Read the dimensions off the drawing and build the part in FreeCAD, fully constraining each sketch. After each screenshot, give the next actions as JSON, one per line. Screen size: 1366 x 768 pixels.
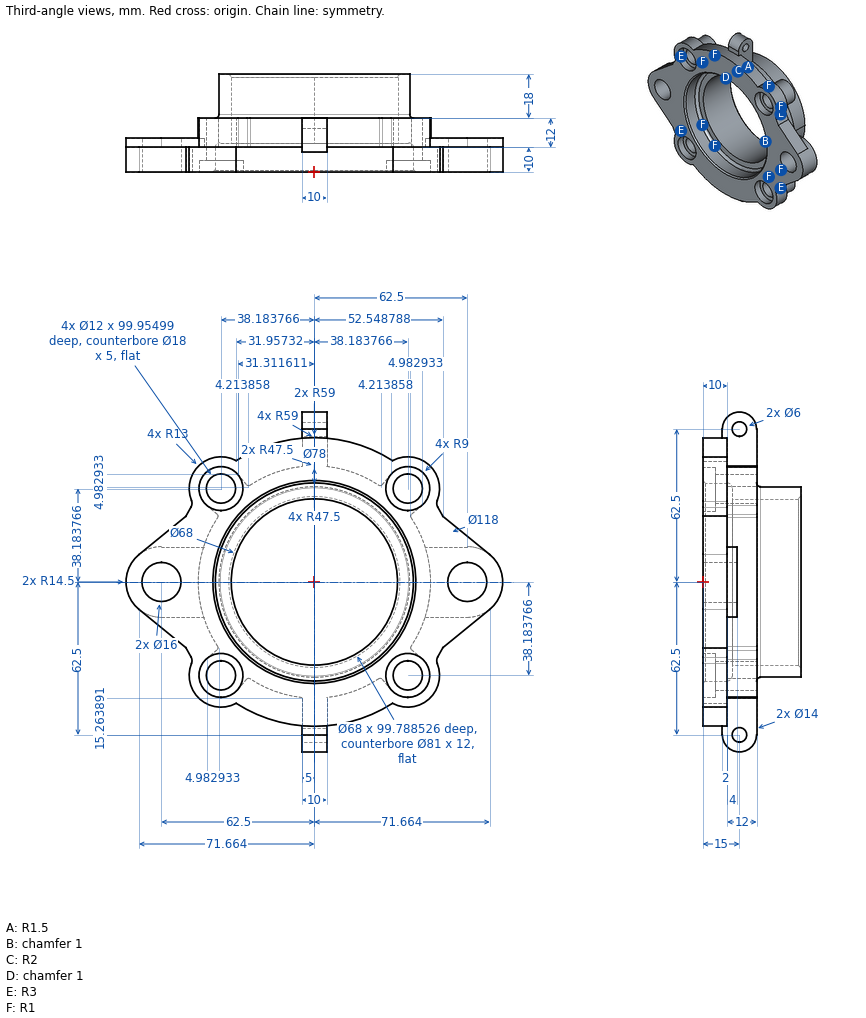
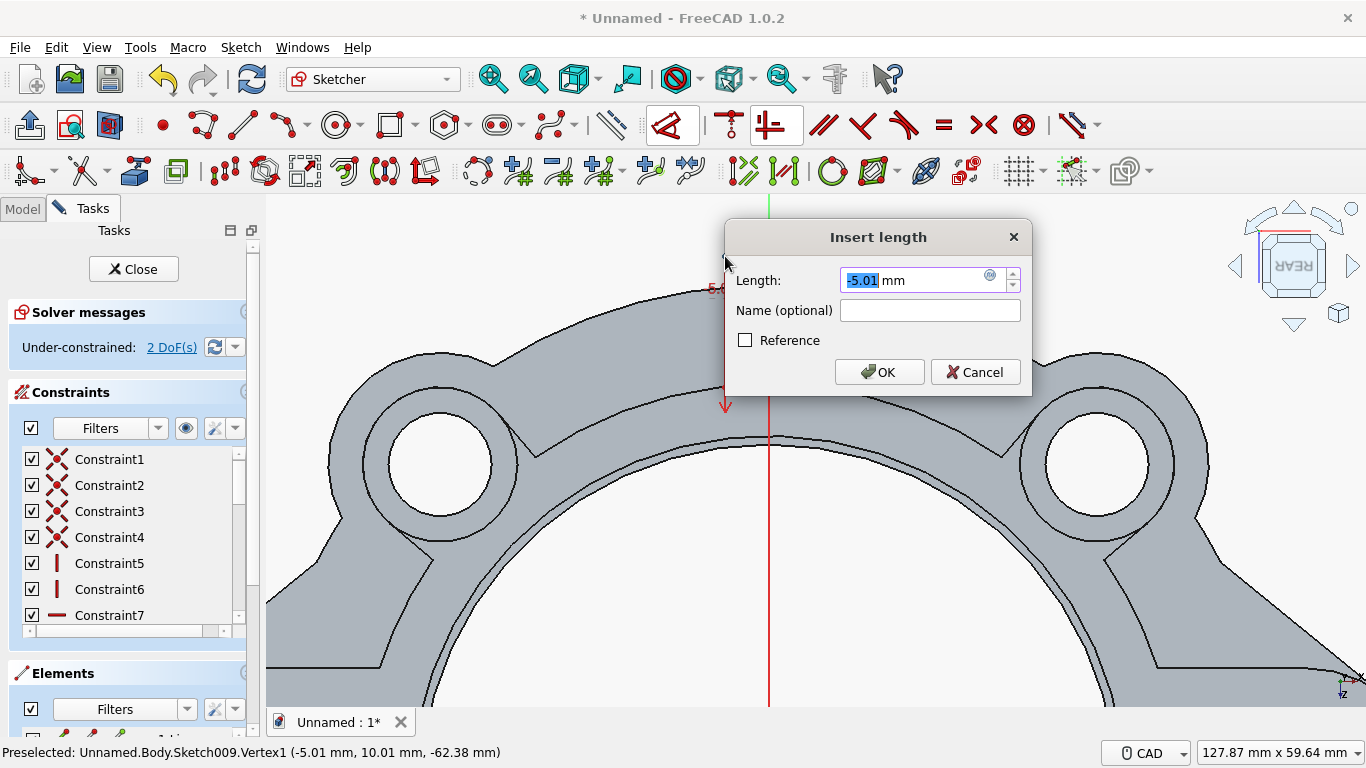
{"action": "type", "text": "-5"}
{"action": "key", "text": "Return"}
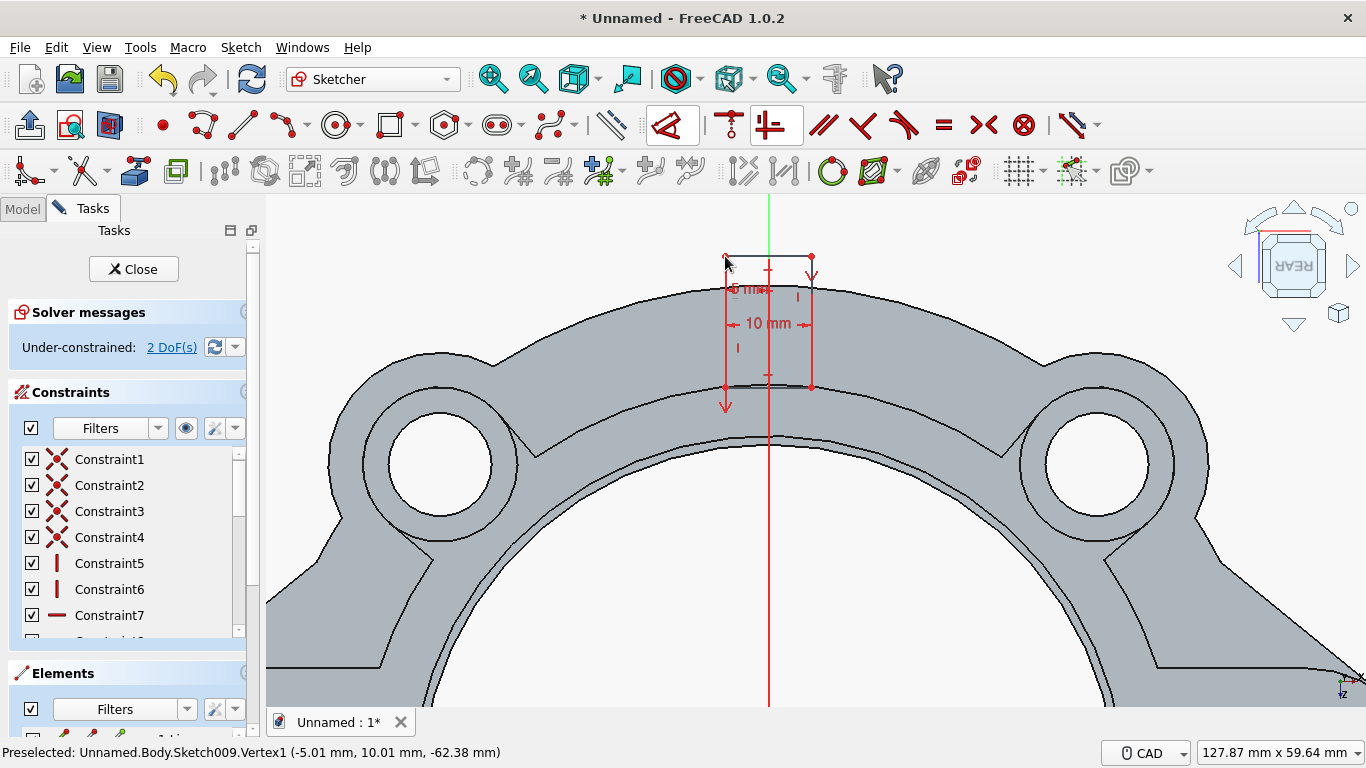
{"action": "left_click", "coordinate": [726, 256]}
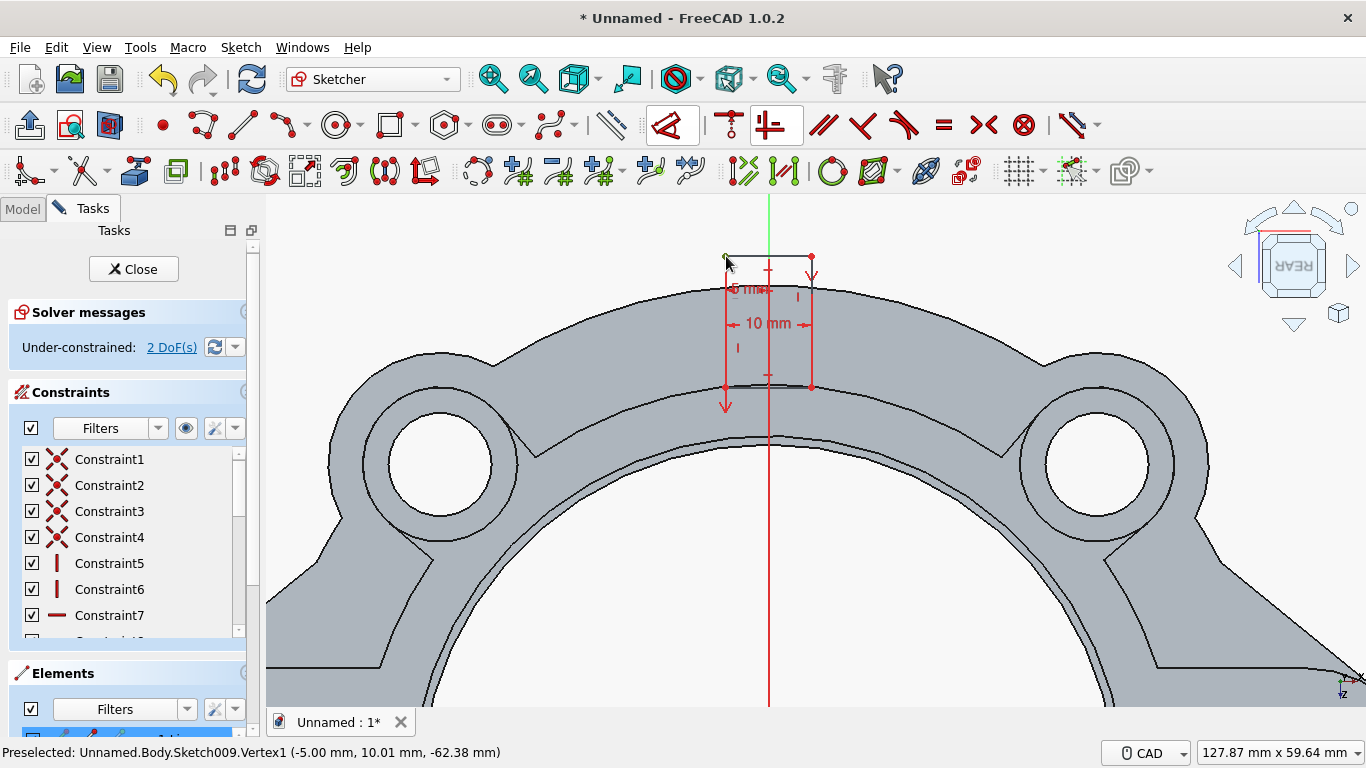
{"action": "left_click", "coordinate": [694, 126]}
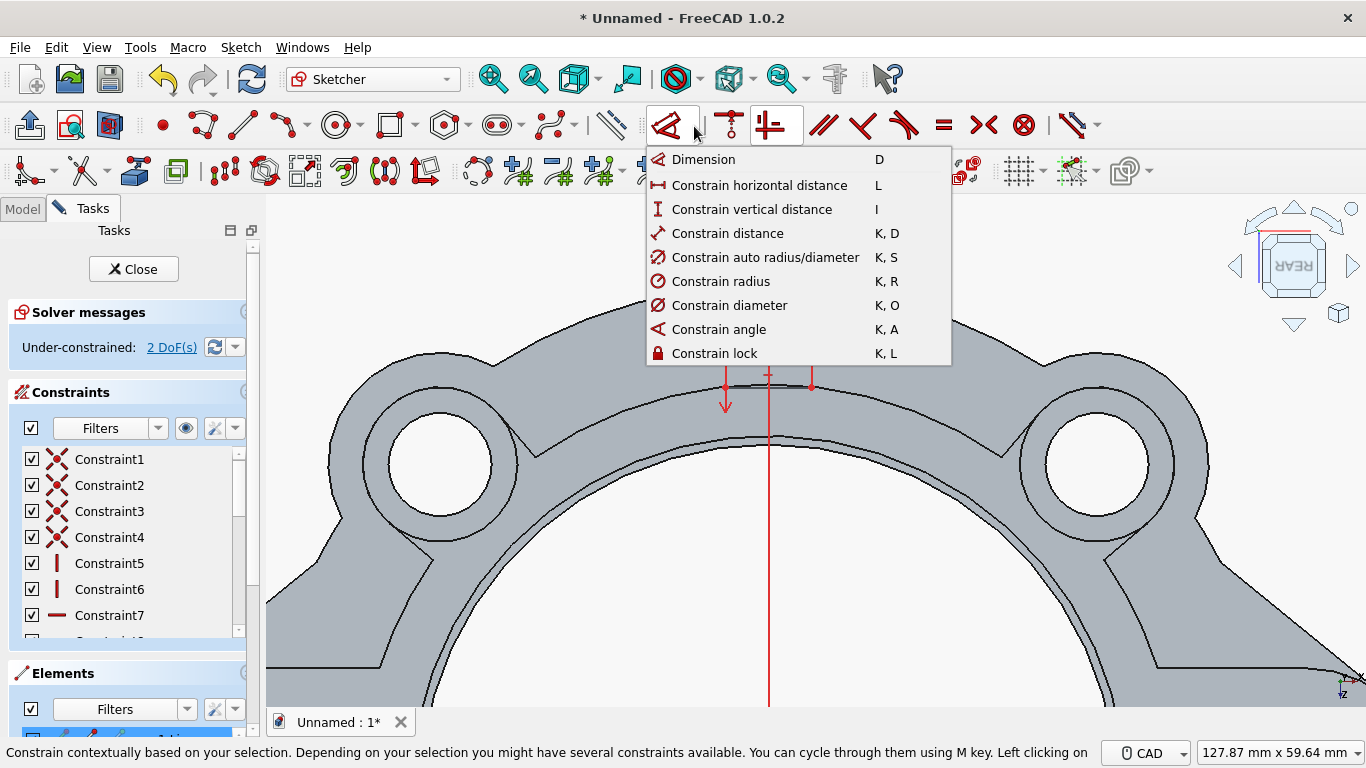
{"action": "left_click", "coordinate": [799, 209]}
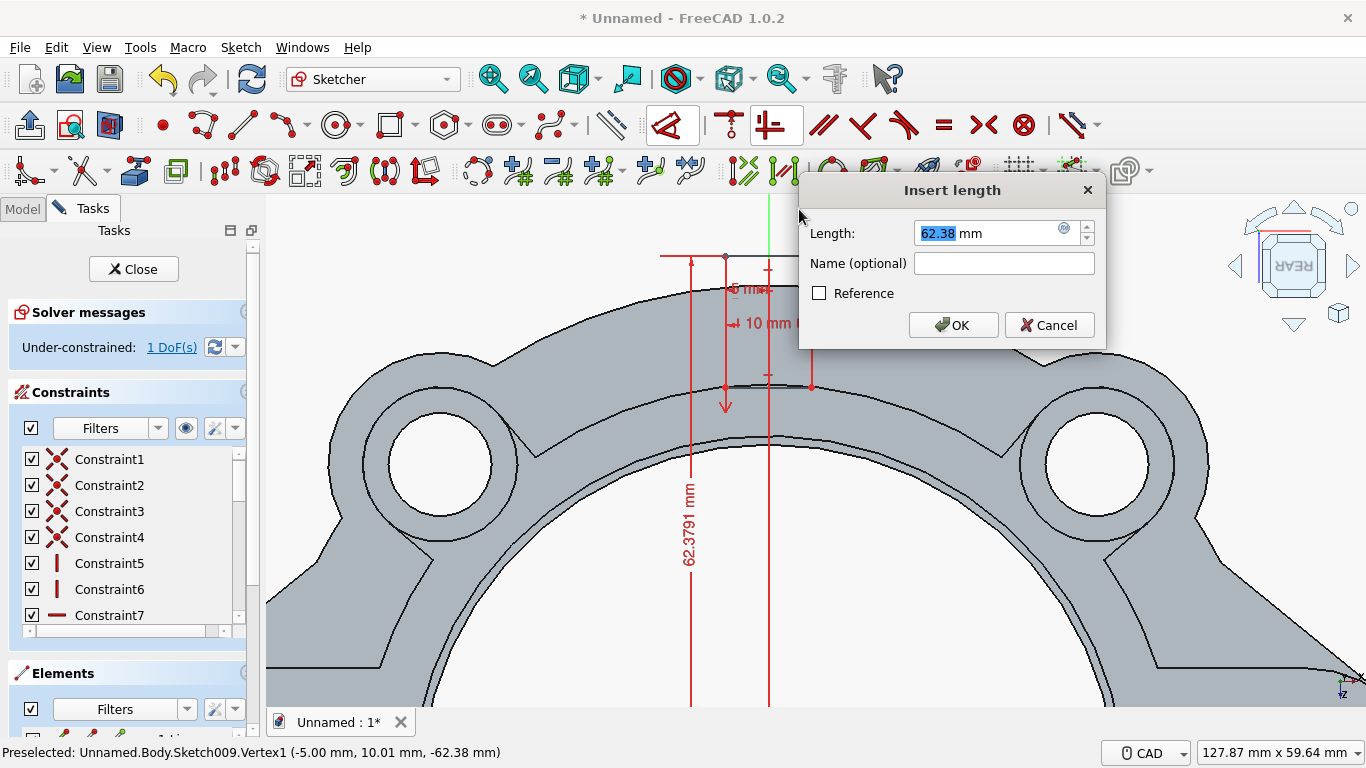
{"action": "type", "text": "62.5"}
{"action": "key", "text": "Return"}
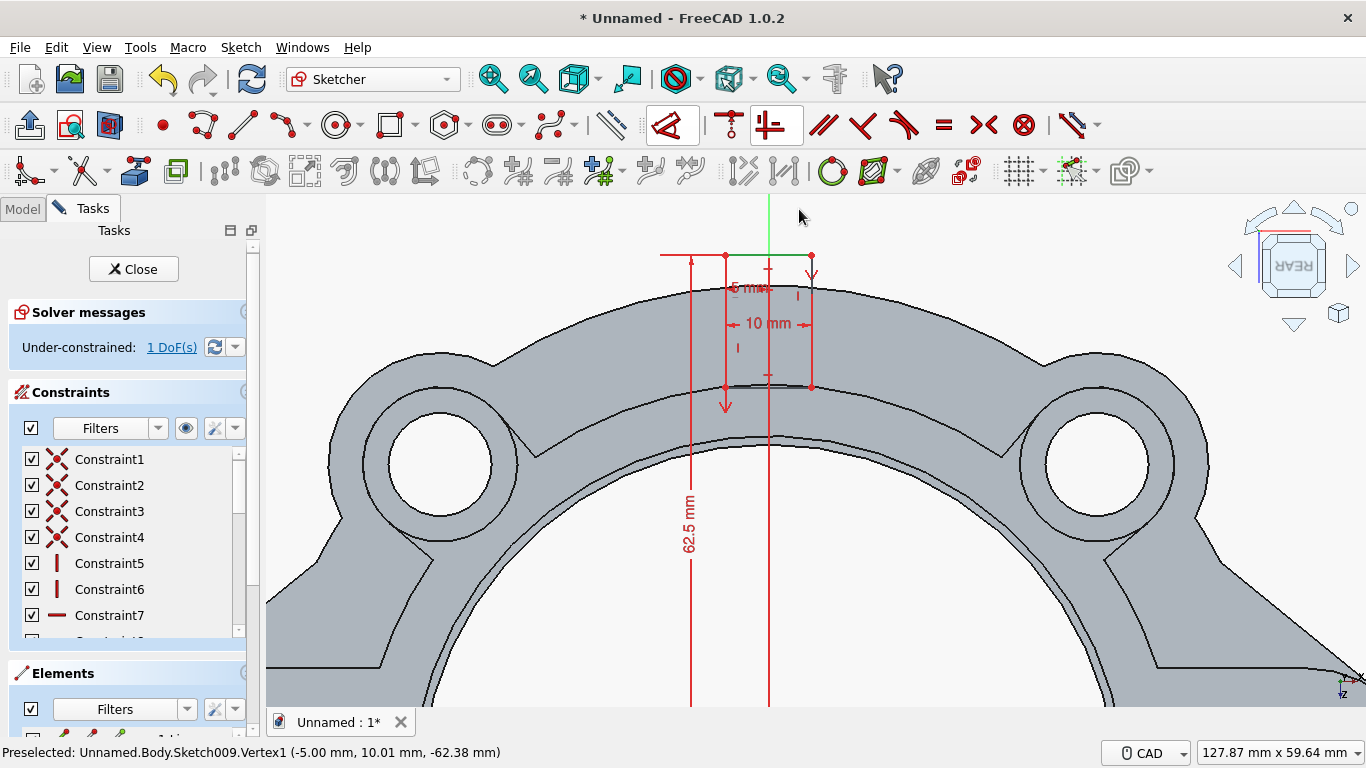
{"action": "left_click", "coordinate": [726, 295]}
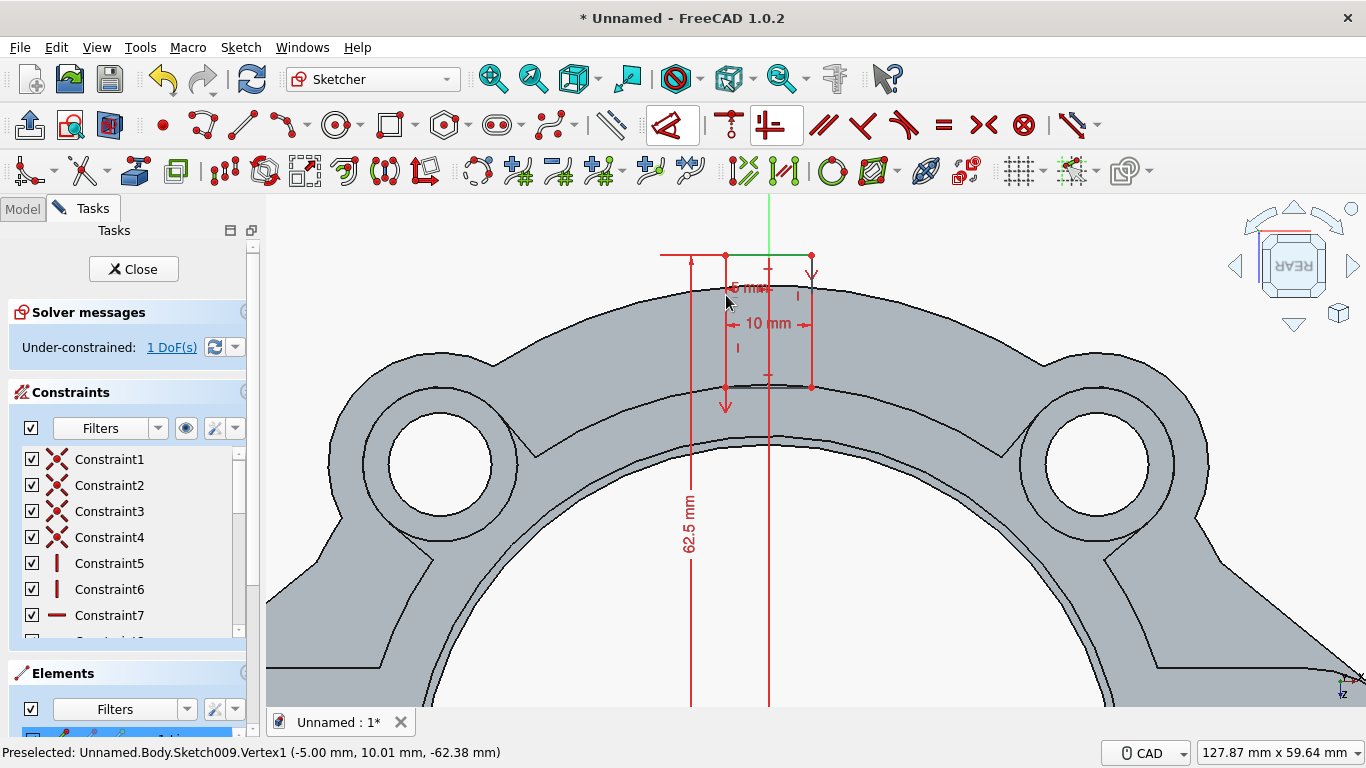
{"action": "key", "text": "i"}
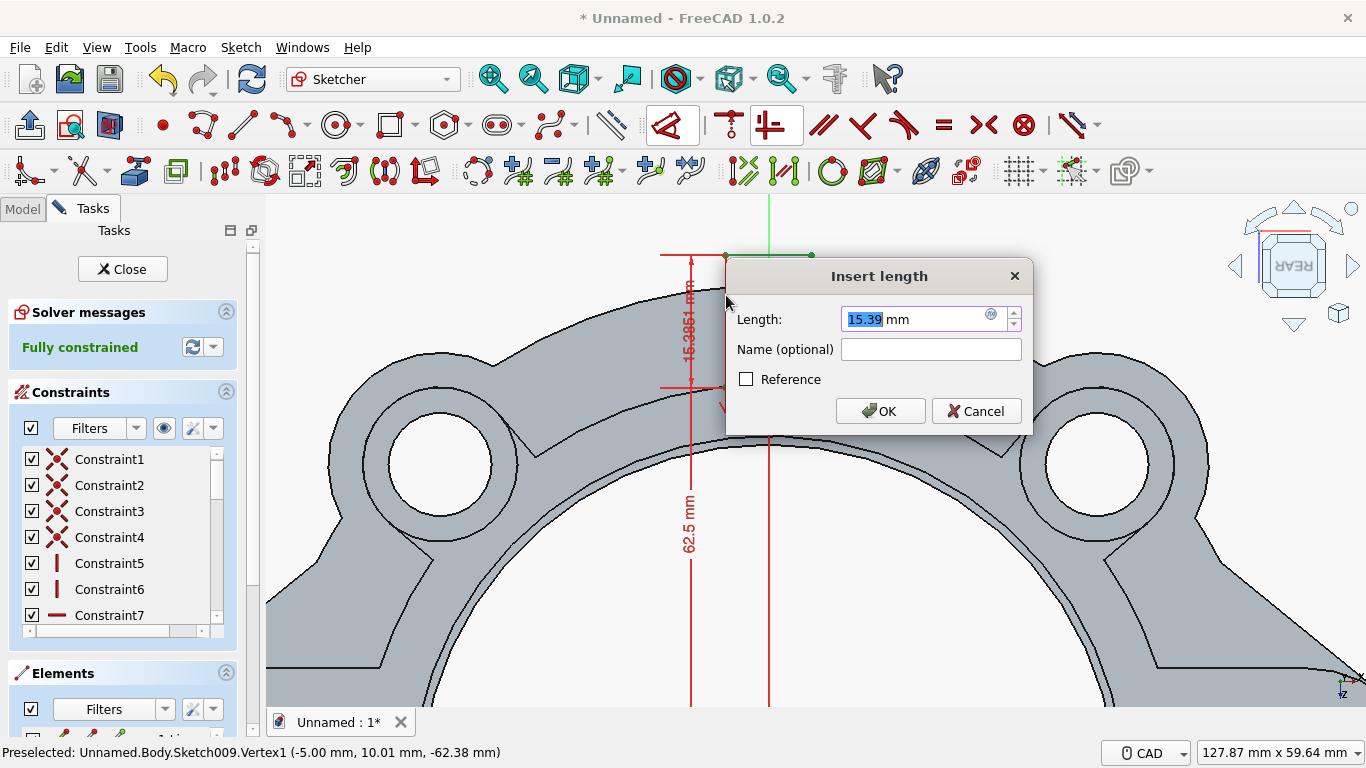
{"action": "type", "text": "15.263891"}
{"action": "key", "text": "Return"}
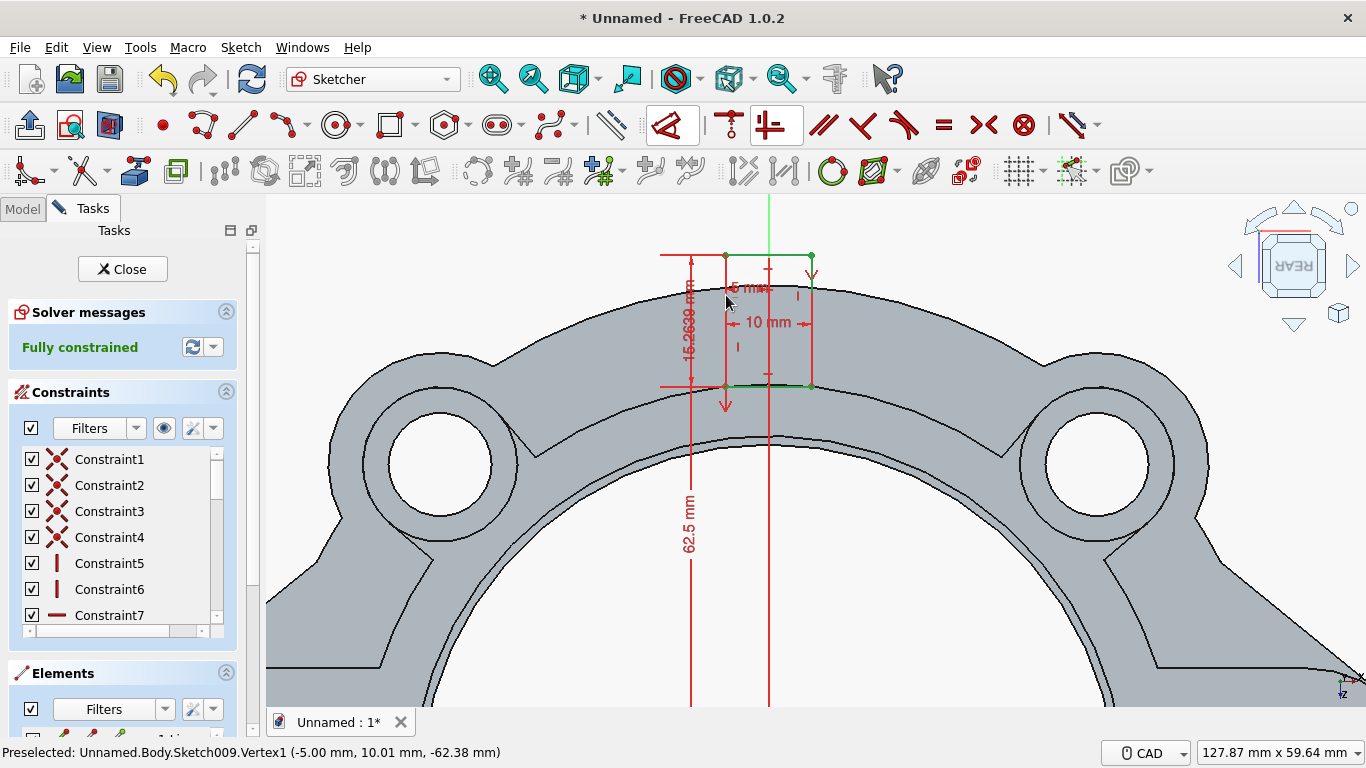
{"action": "left_click", "coordinate": [123, 269]}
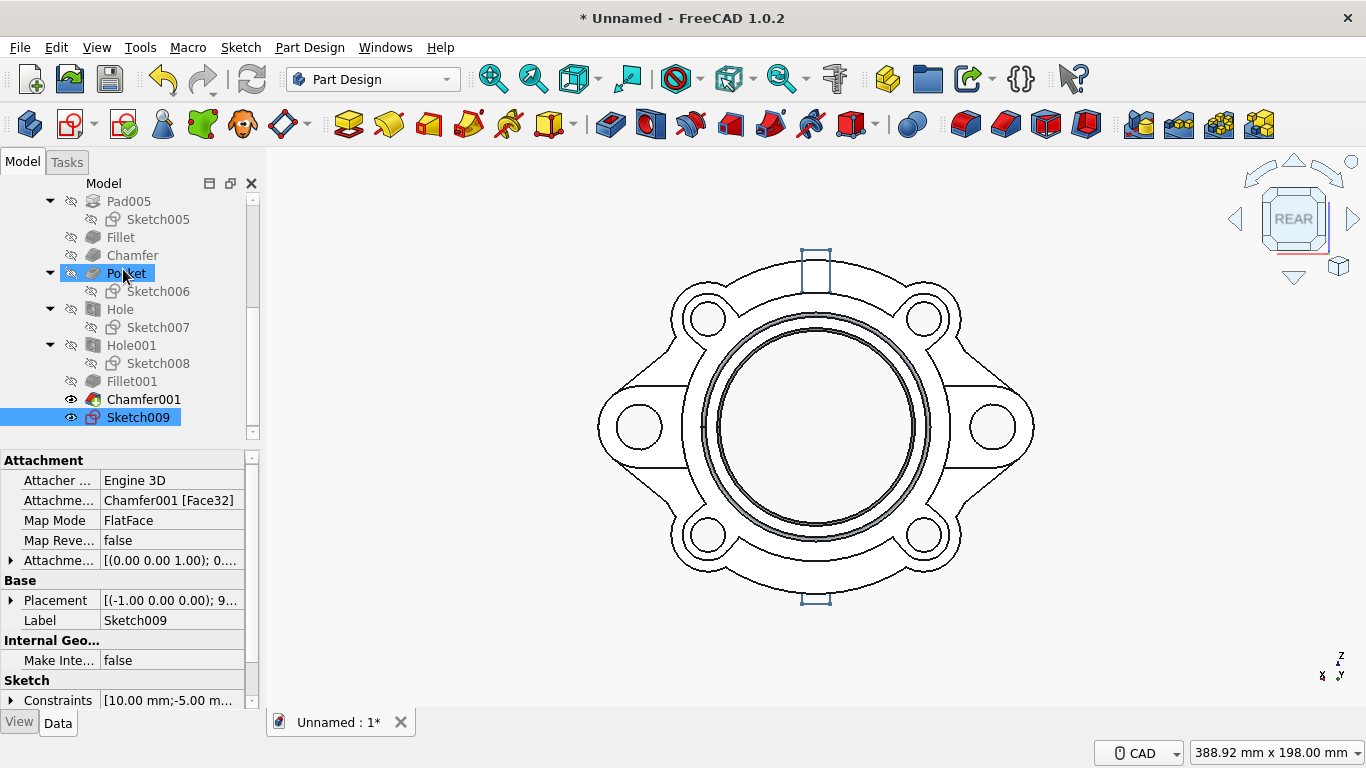
{"action": "left_click", "coordinate": [350, 124]}